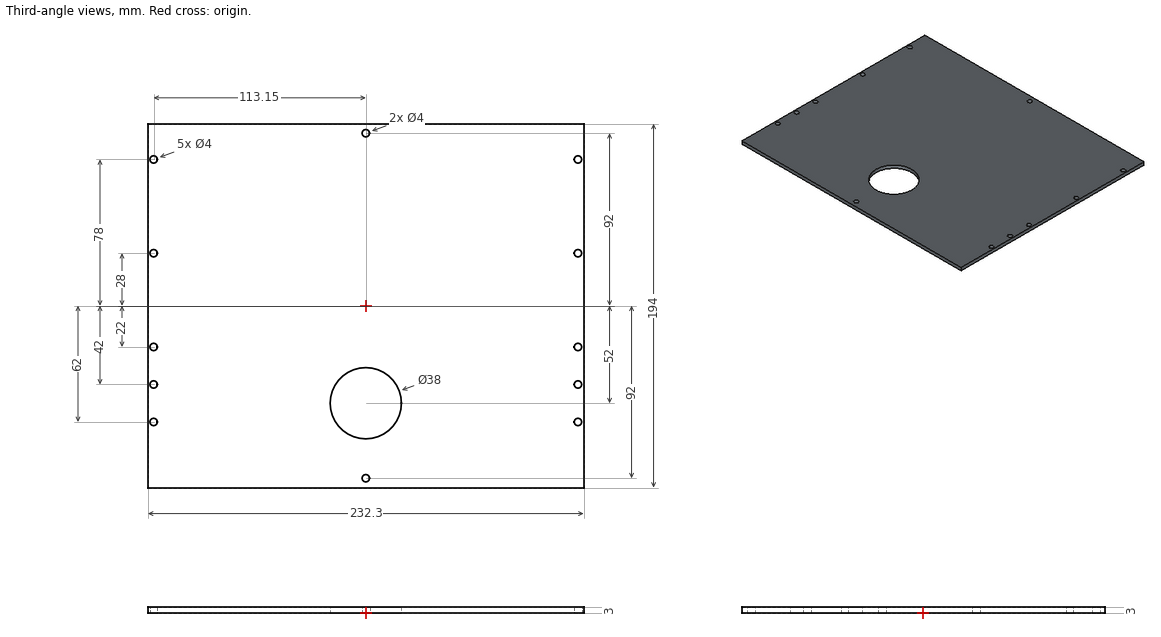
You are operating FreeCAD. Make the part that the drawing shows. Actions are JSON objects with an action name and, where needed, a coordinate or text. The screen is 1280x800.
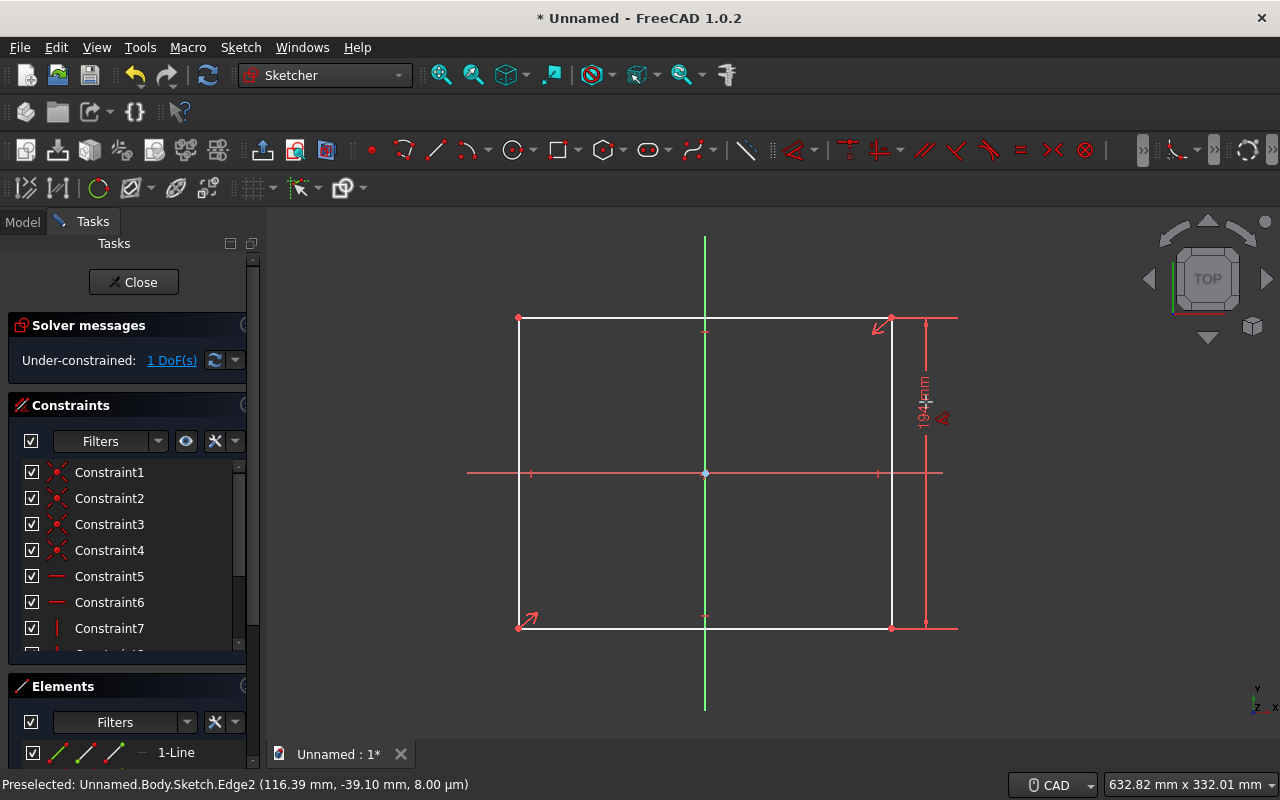
{"action": "left_click", "coordinate": [630, 629]}
{"action": "left_click", "coordinate": [619, 663]}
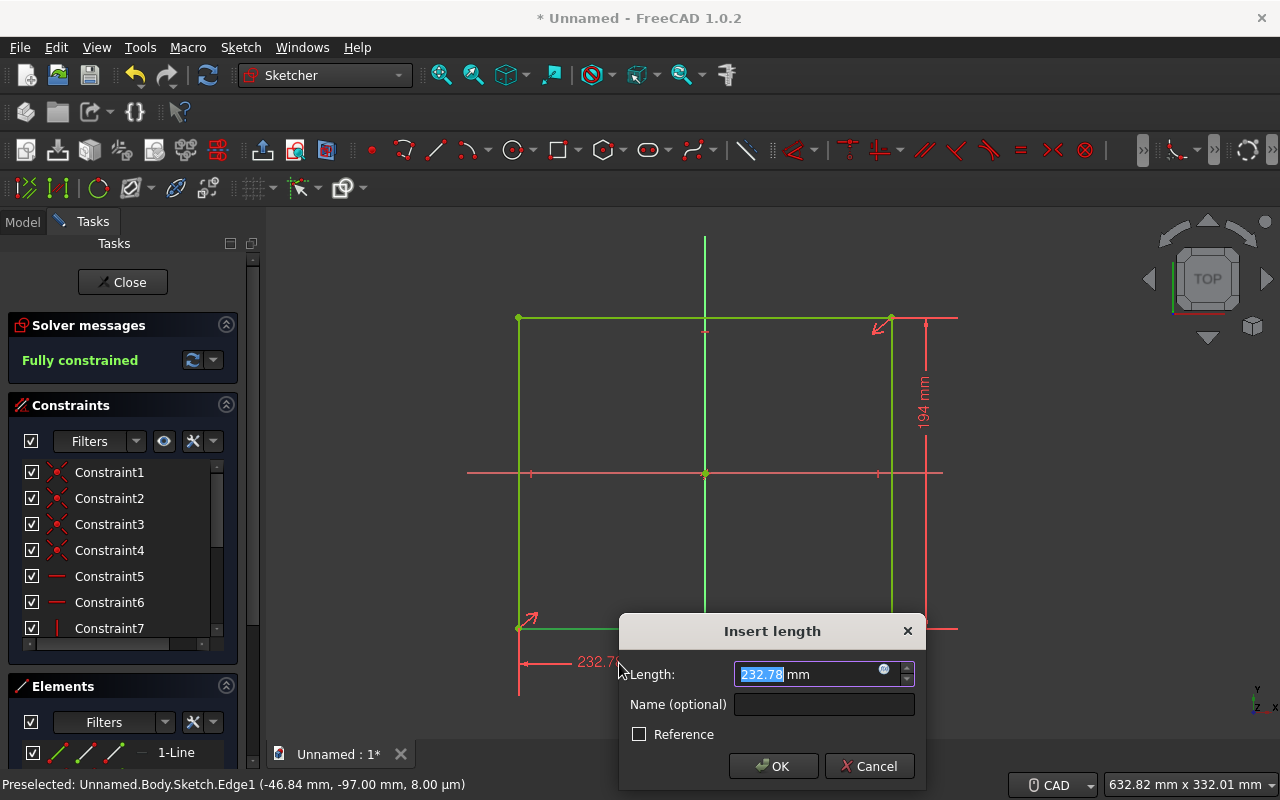
{"action": "type", "text": "232.3"}
{"action": "key", "text": "Return"}
{"action": "key", "text": "Escape"}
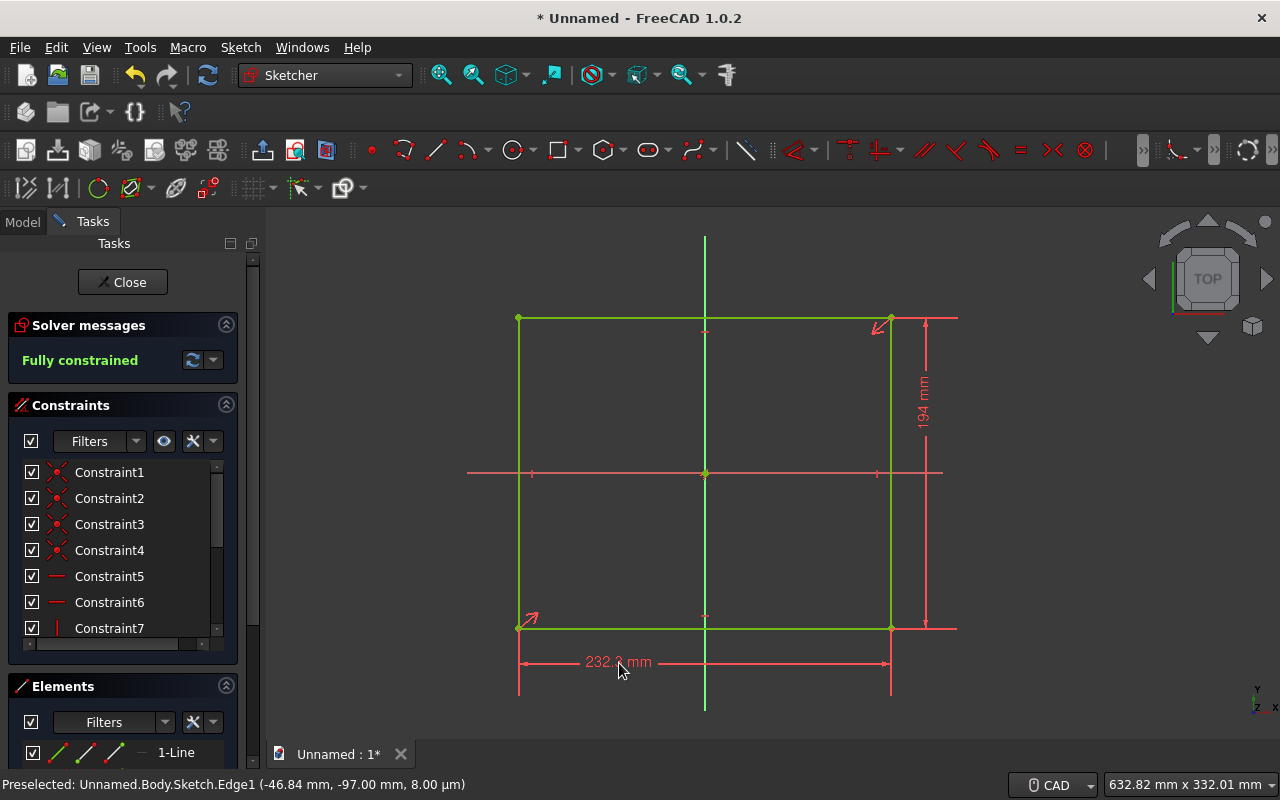
{"action": "left_click", "coordinate": [123, 282]}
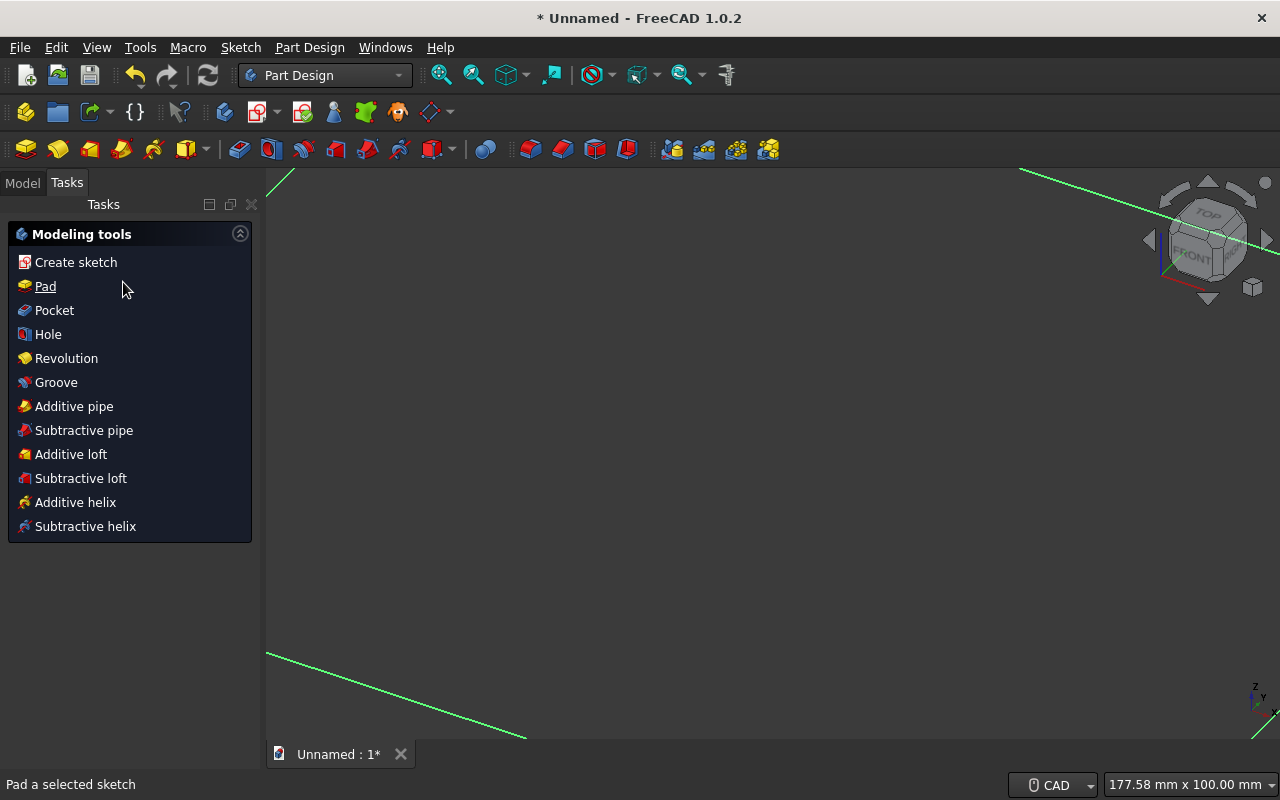
{"action": "left_click", "coordinate": [26, 150]}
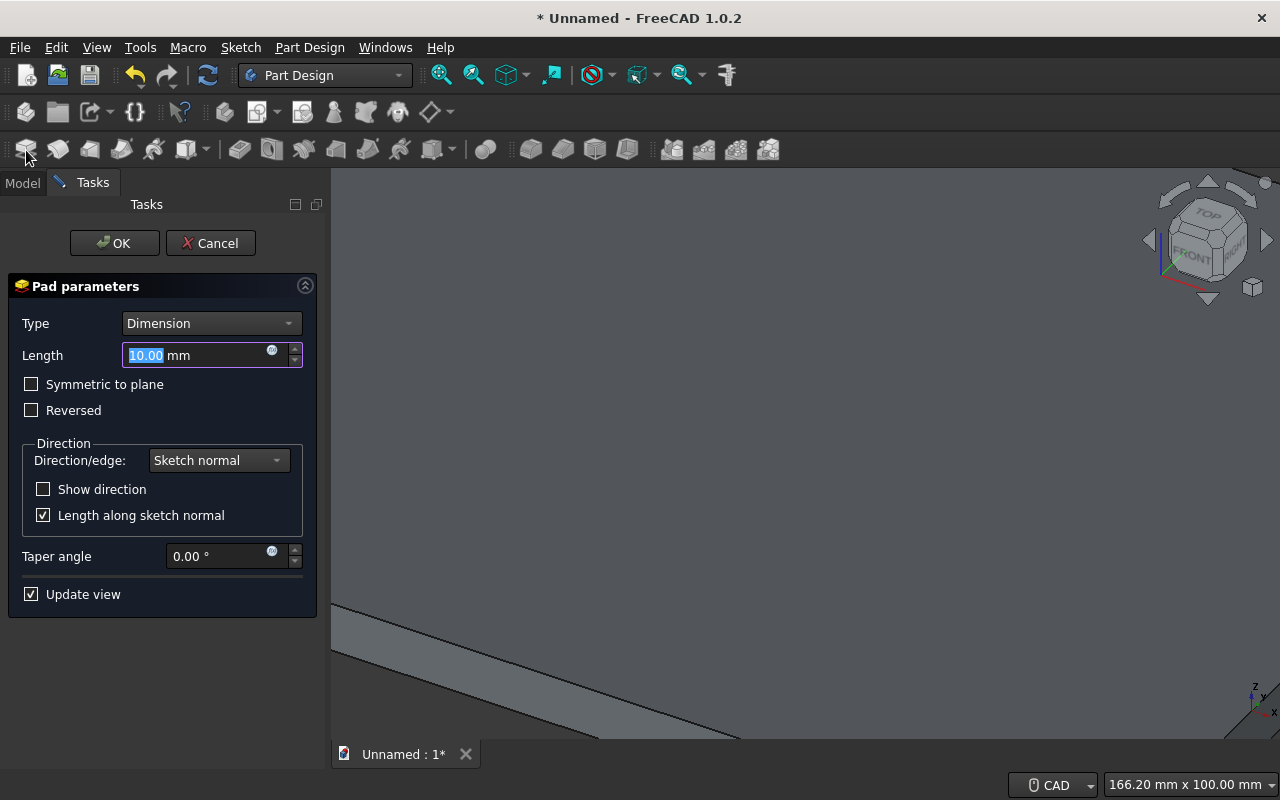
{"action": "type", "text": "3"}
{"action": "key", "text": "Tab"}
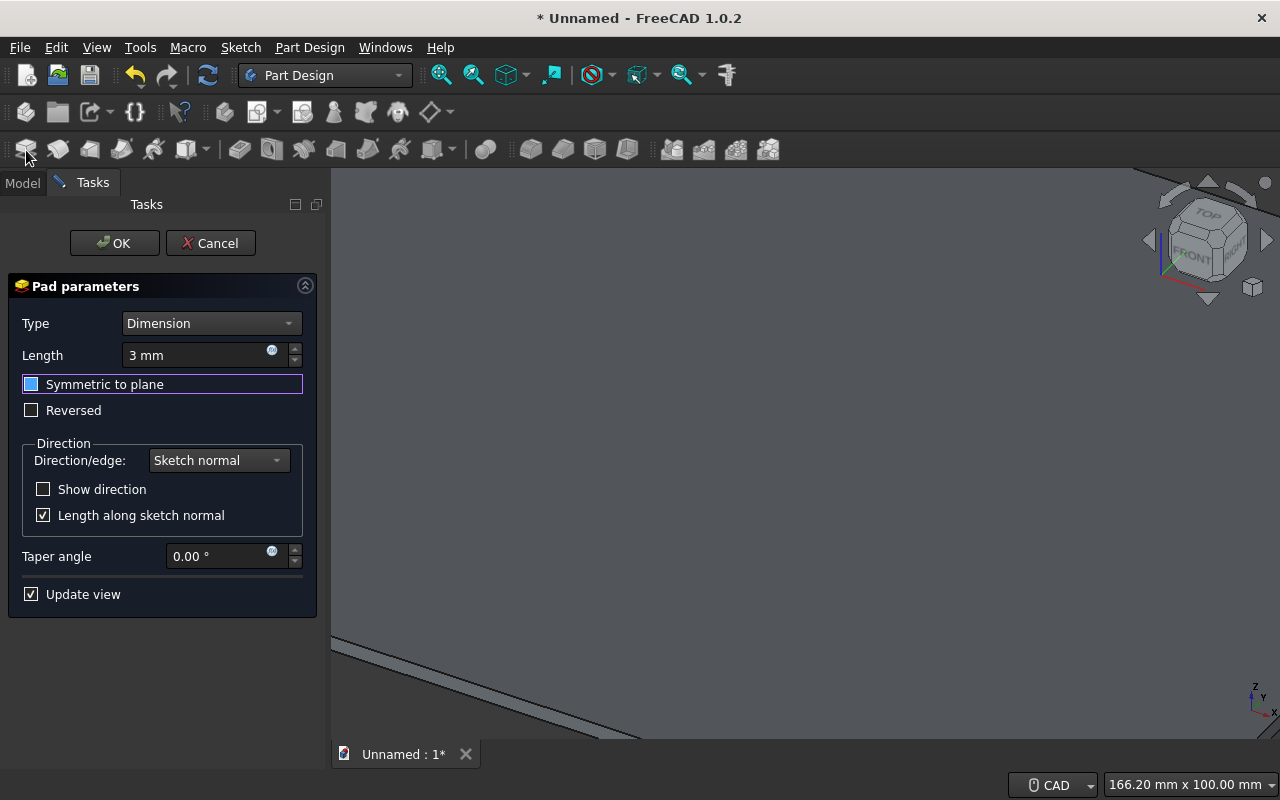
{"action": "left_click", "coordinate": [115, 243]}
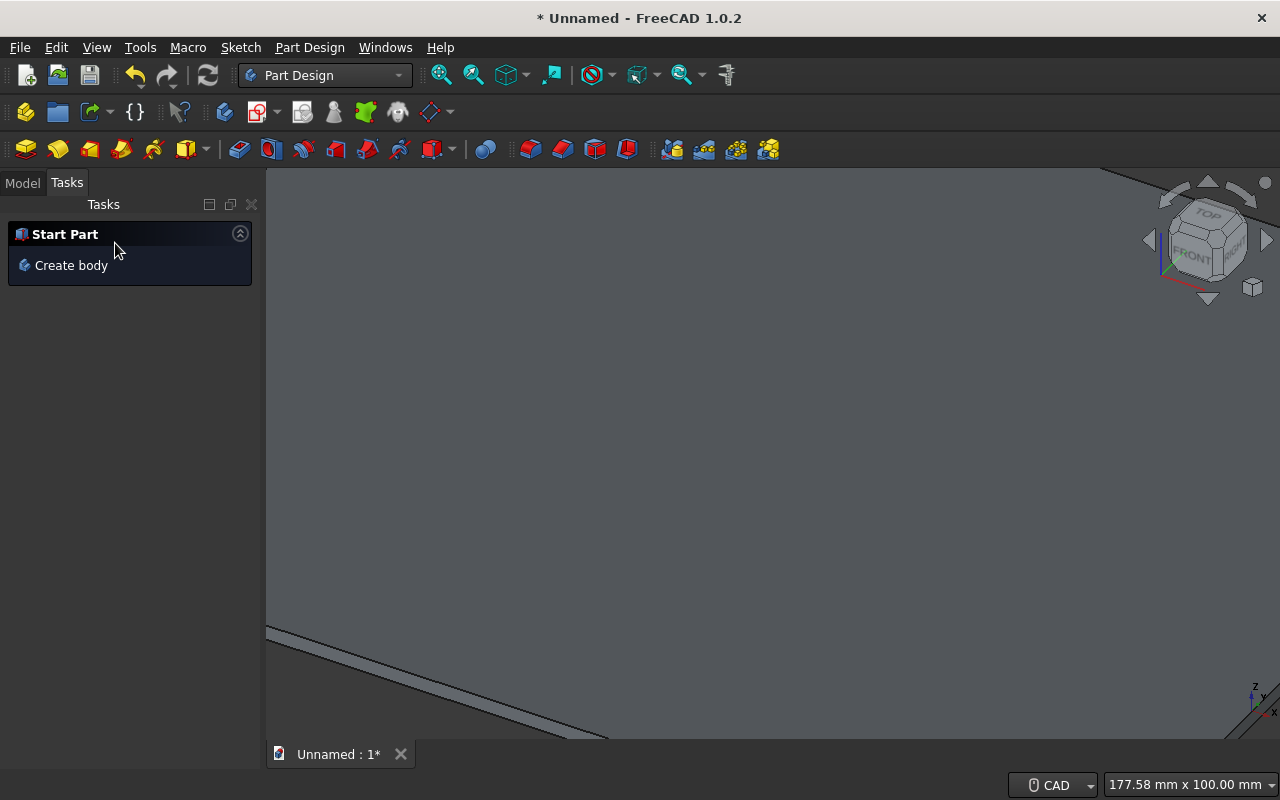
{"action": "left_click", "coordinate": [442, 76]}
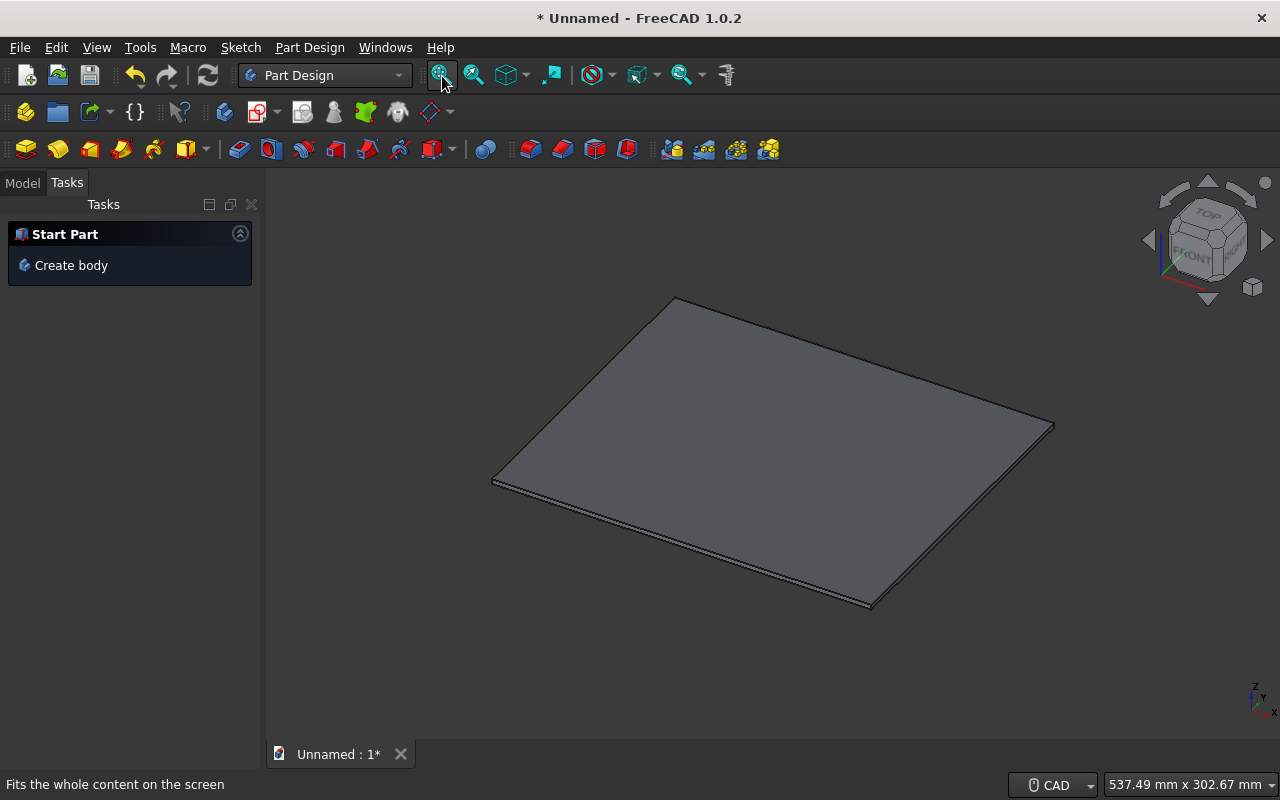
{"action": "left_click", "coordinate": [773, 450]}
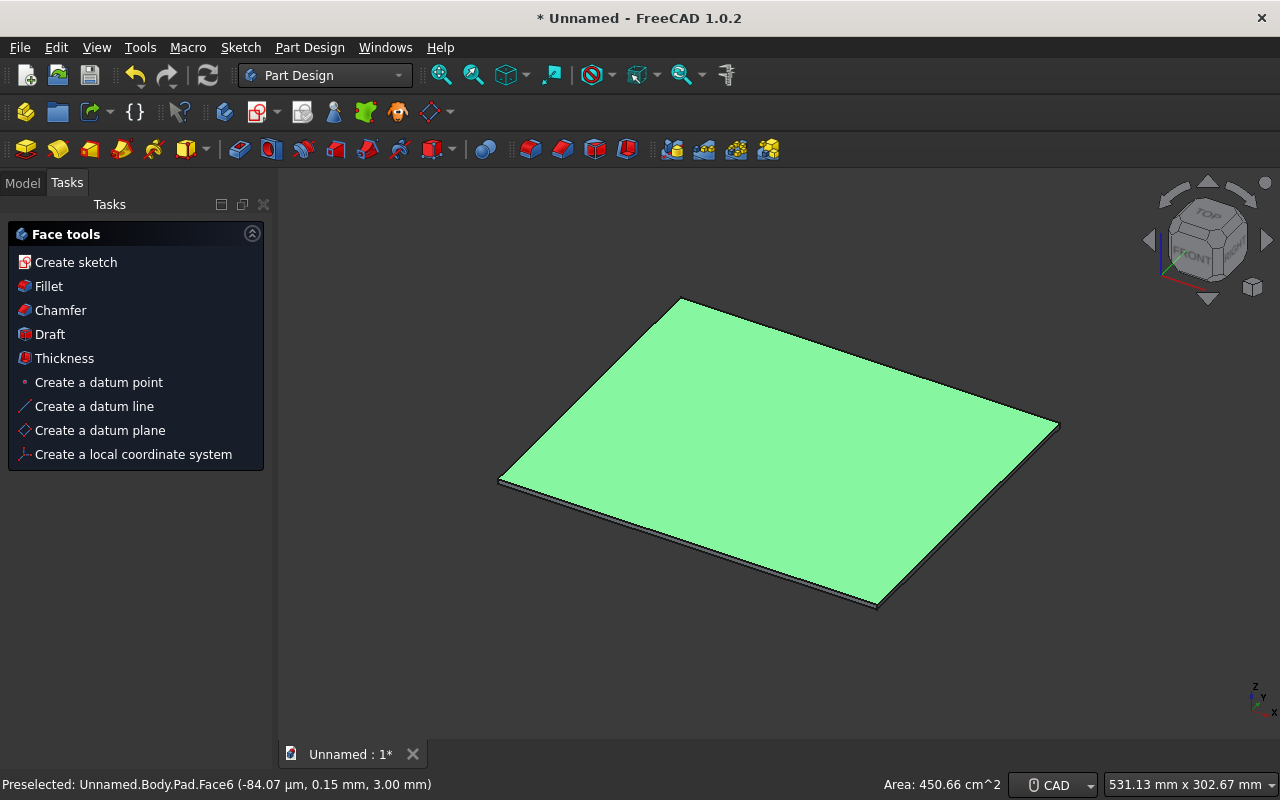
{"action": "left_click", "coordinate": [258, 112]}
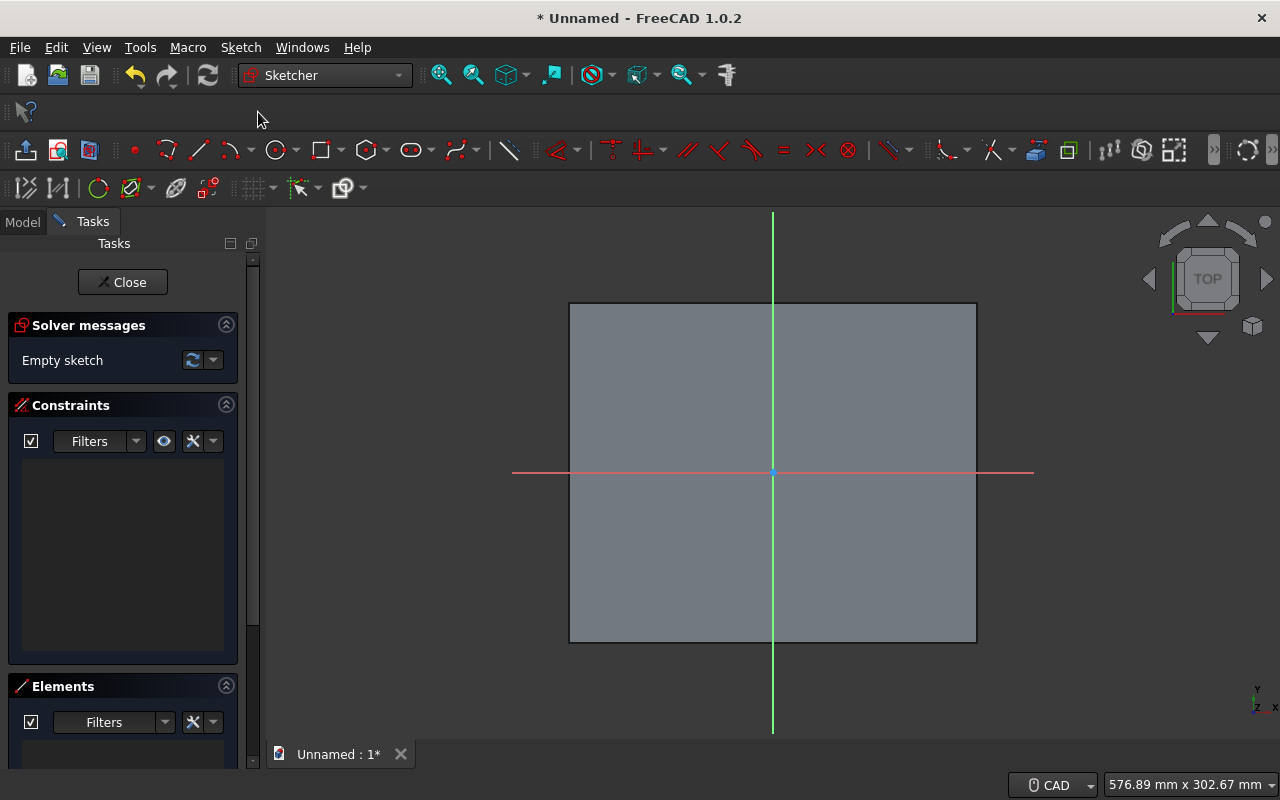
{"action": "scroll", "coordinate": [813, 572], "scroll_direction": "up", "scroll_amount": 5}